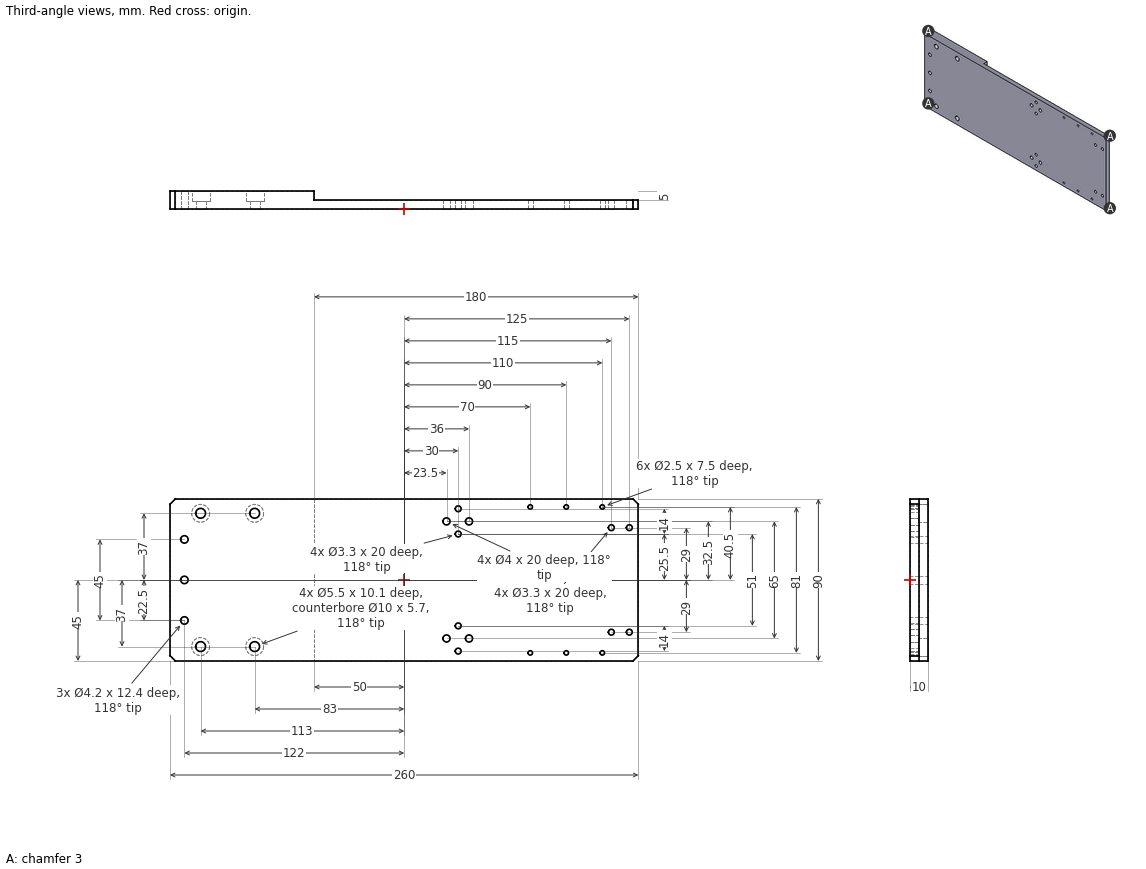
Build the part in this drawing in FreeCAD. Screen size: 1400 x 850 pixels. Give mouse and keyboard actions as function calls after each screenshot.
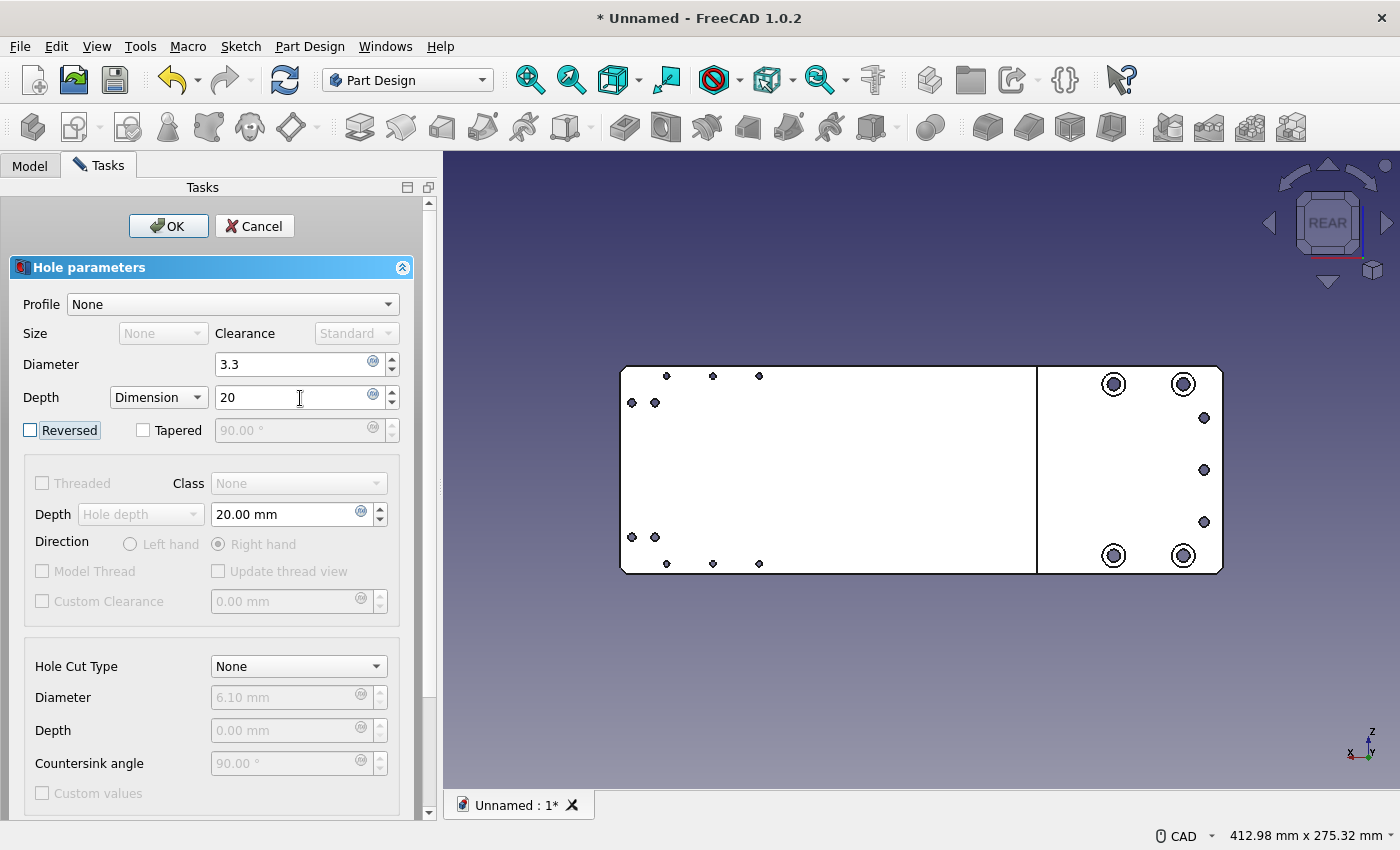
click(169, 226)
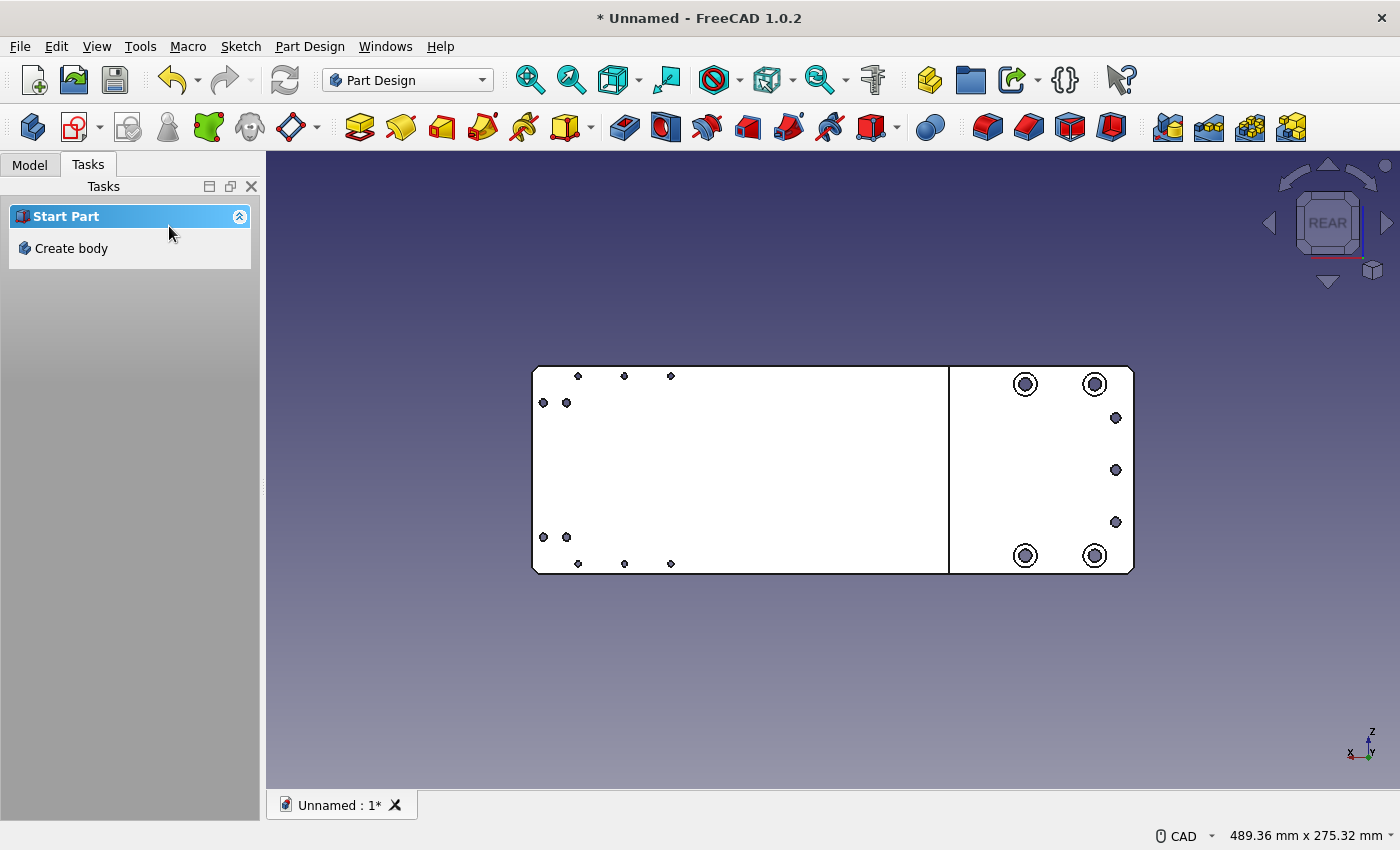
click(1042, 469)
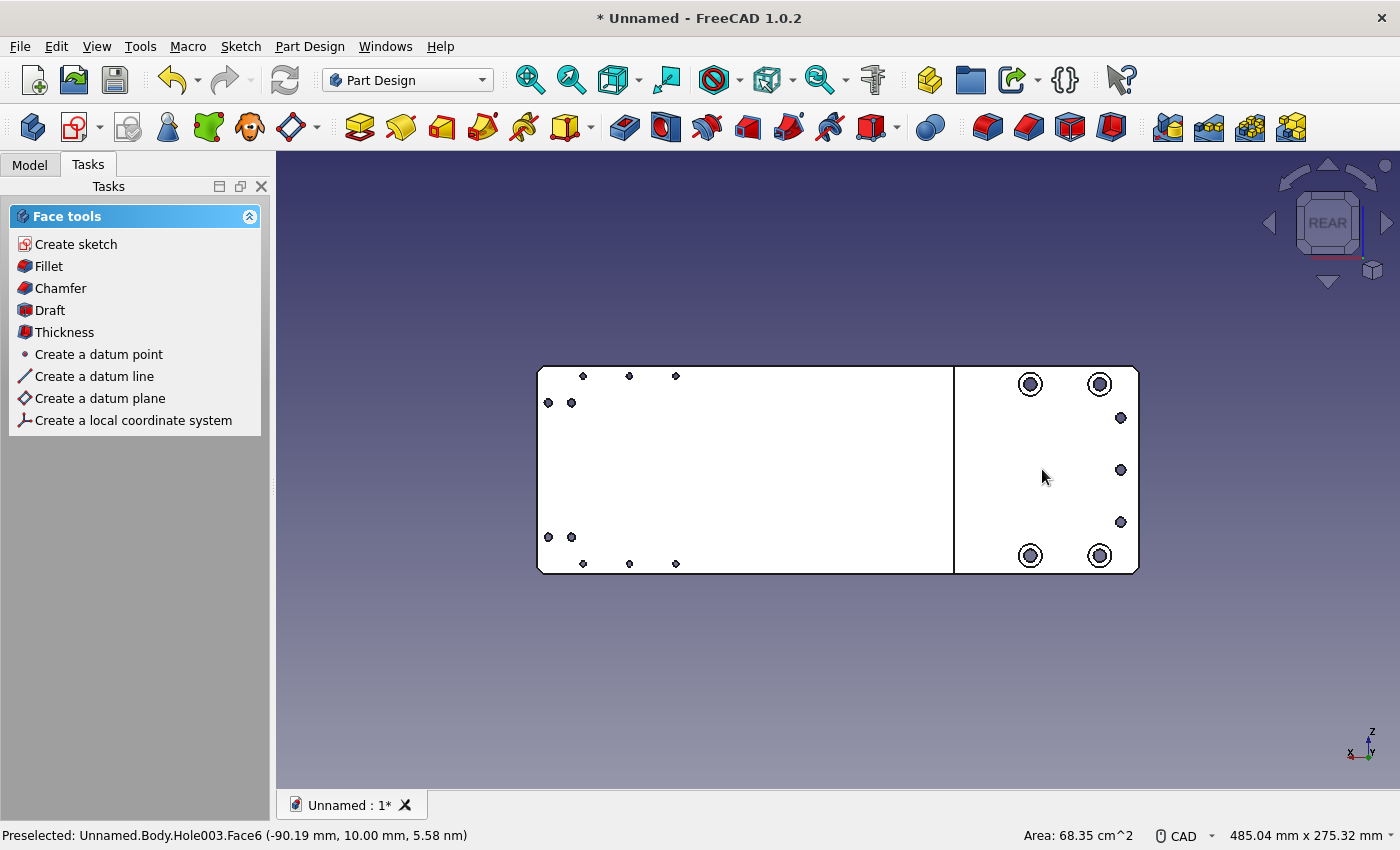
click(74, 128)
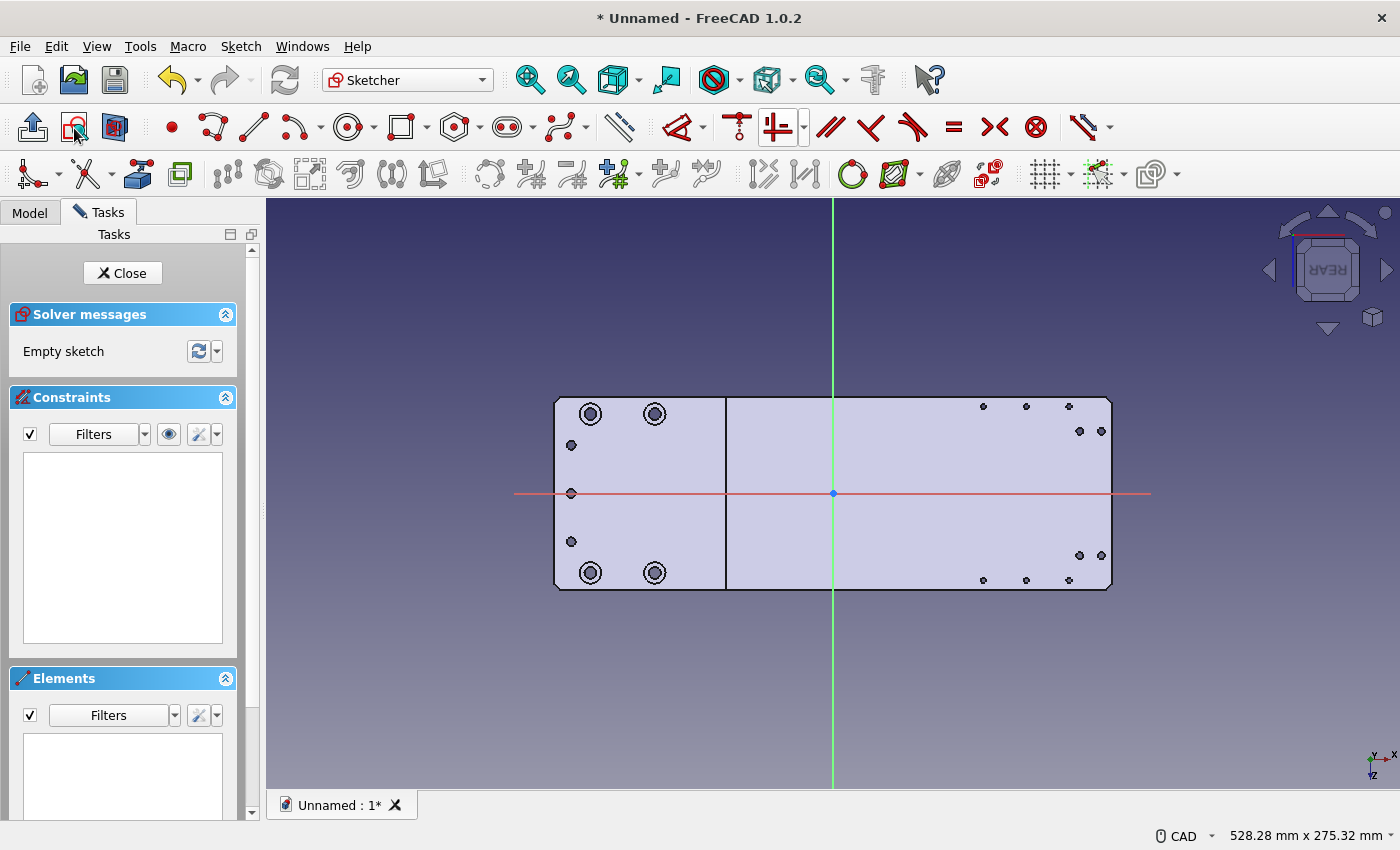
scroll(951, 493, up, 4)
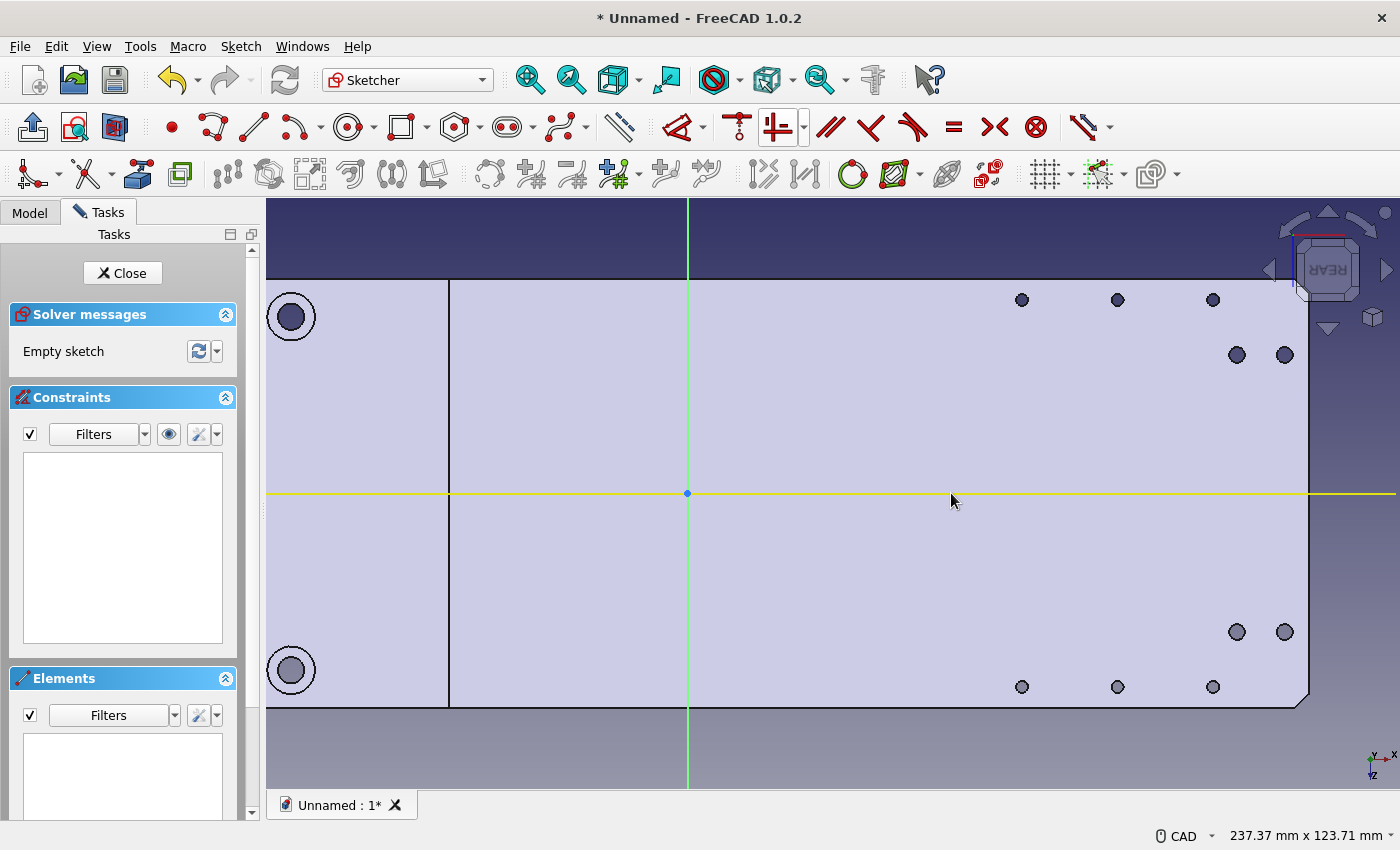
click(348, 128)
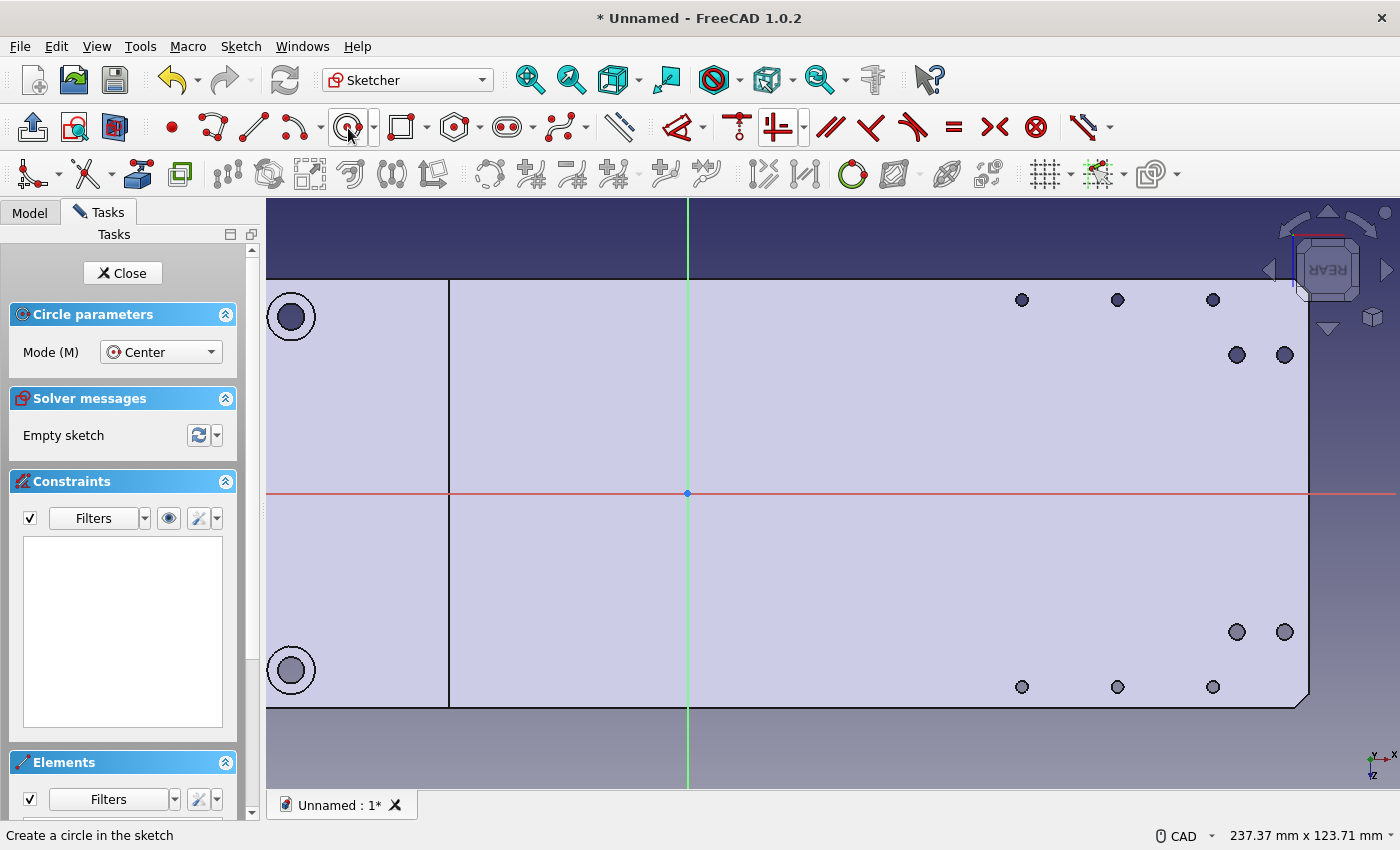
scroll(831, 615, up, 6)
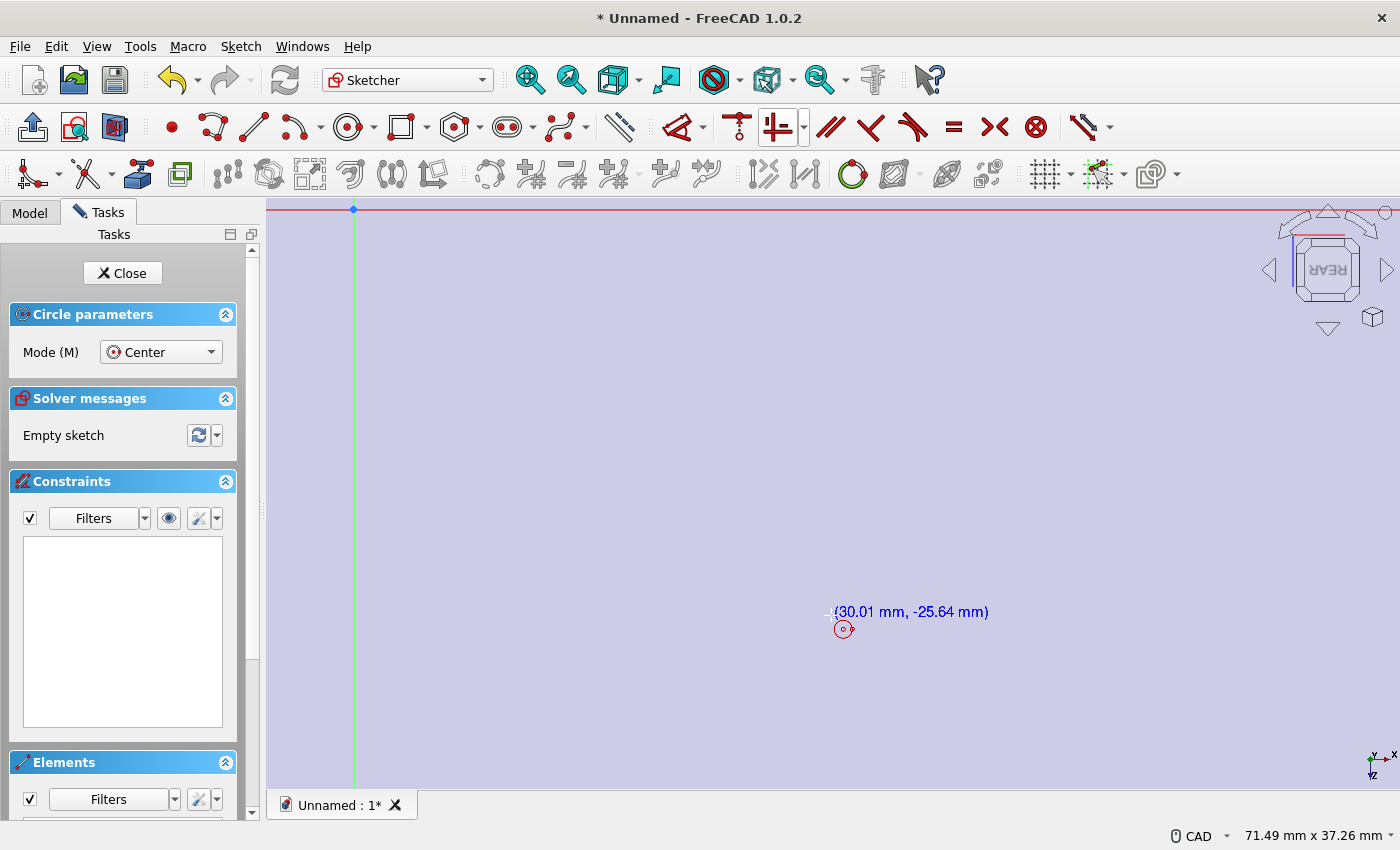
click(830, 614)
click(848, 596)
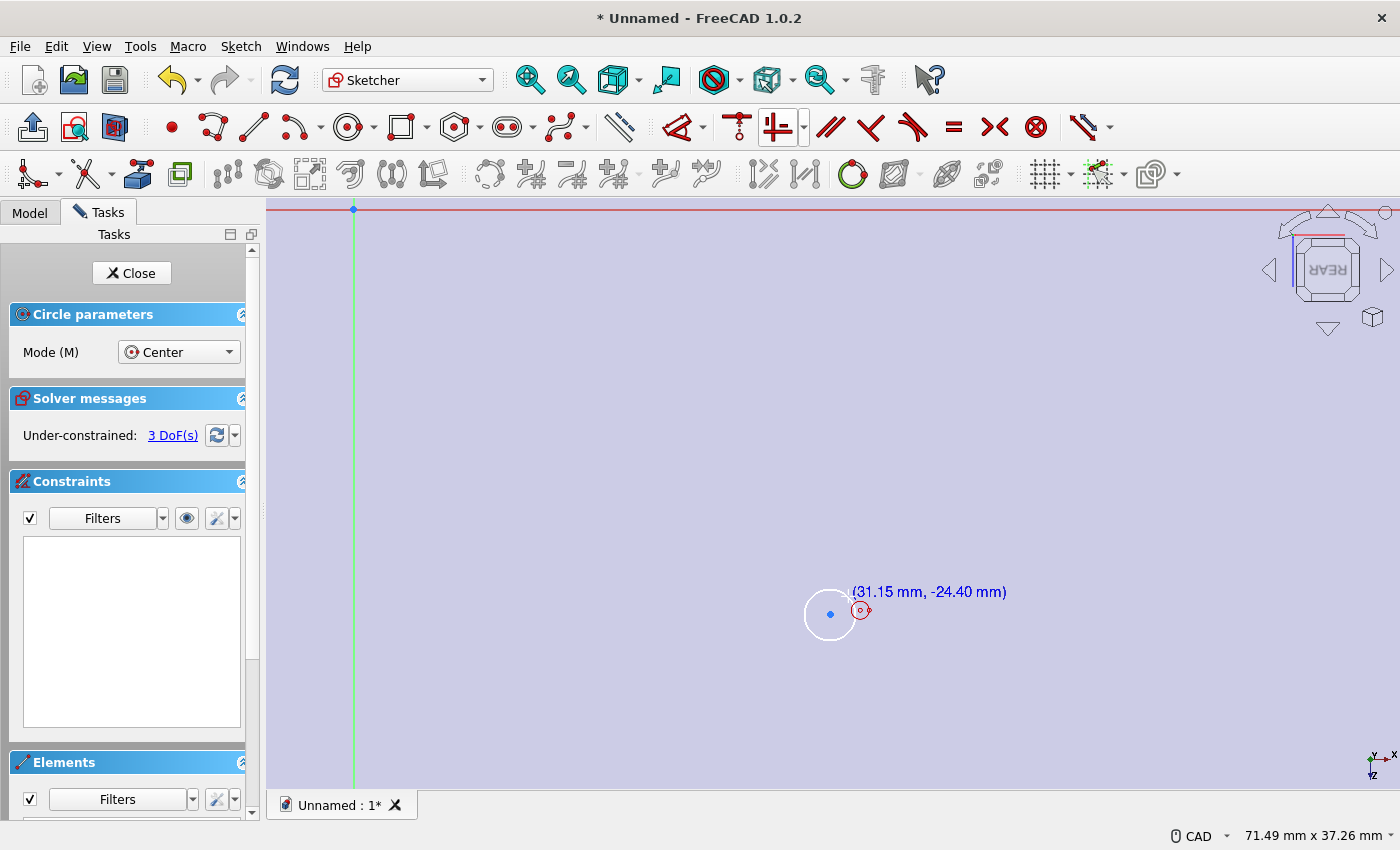
scroll(833, 616, down, 6)